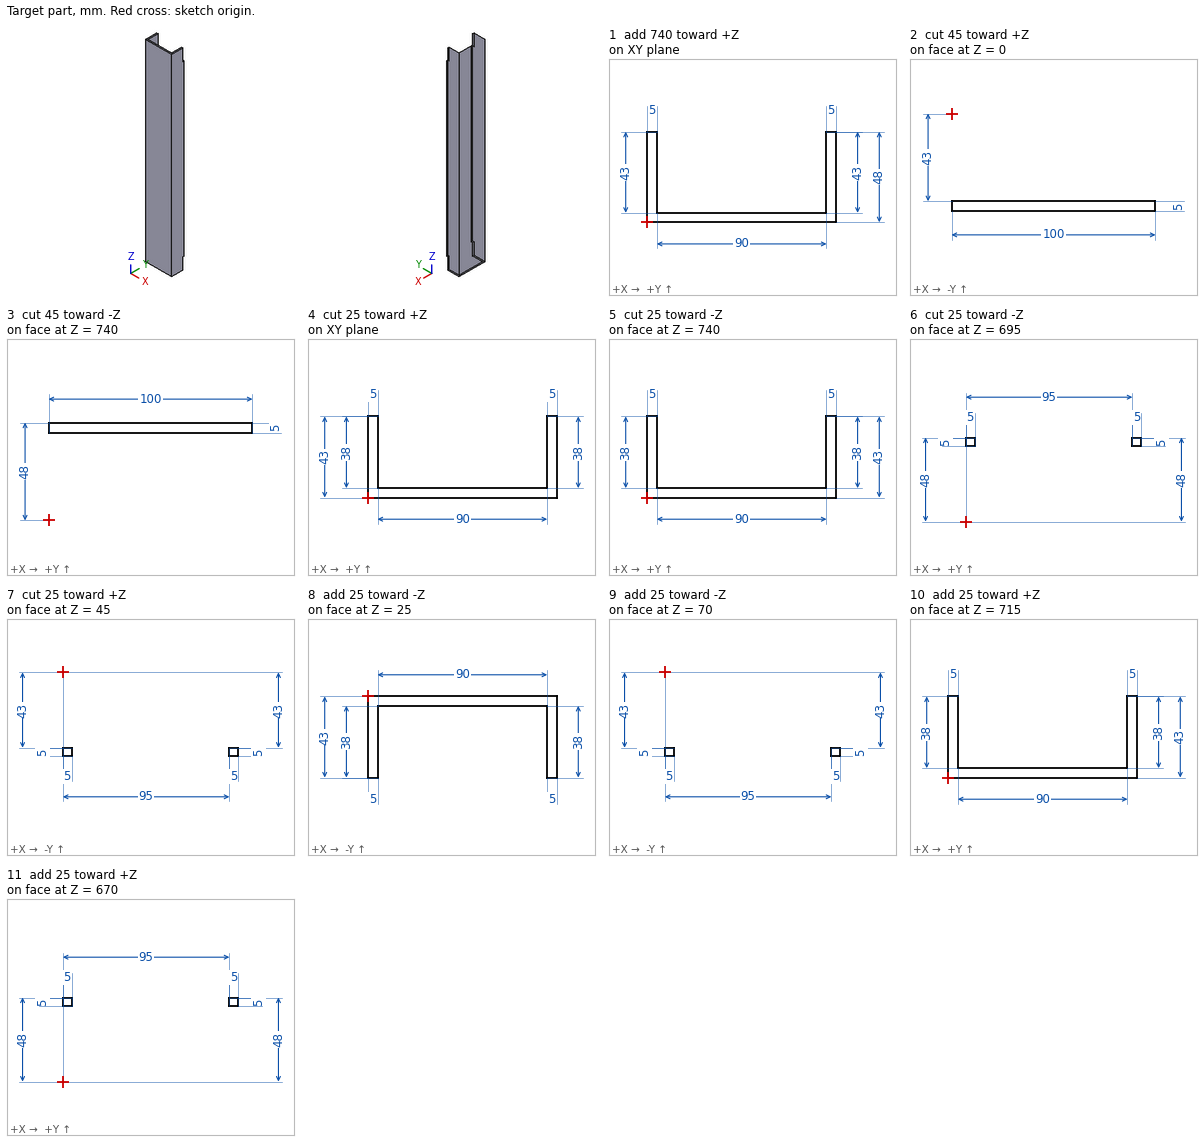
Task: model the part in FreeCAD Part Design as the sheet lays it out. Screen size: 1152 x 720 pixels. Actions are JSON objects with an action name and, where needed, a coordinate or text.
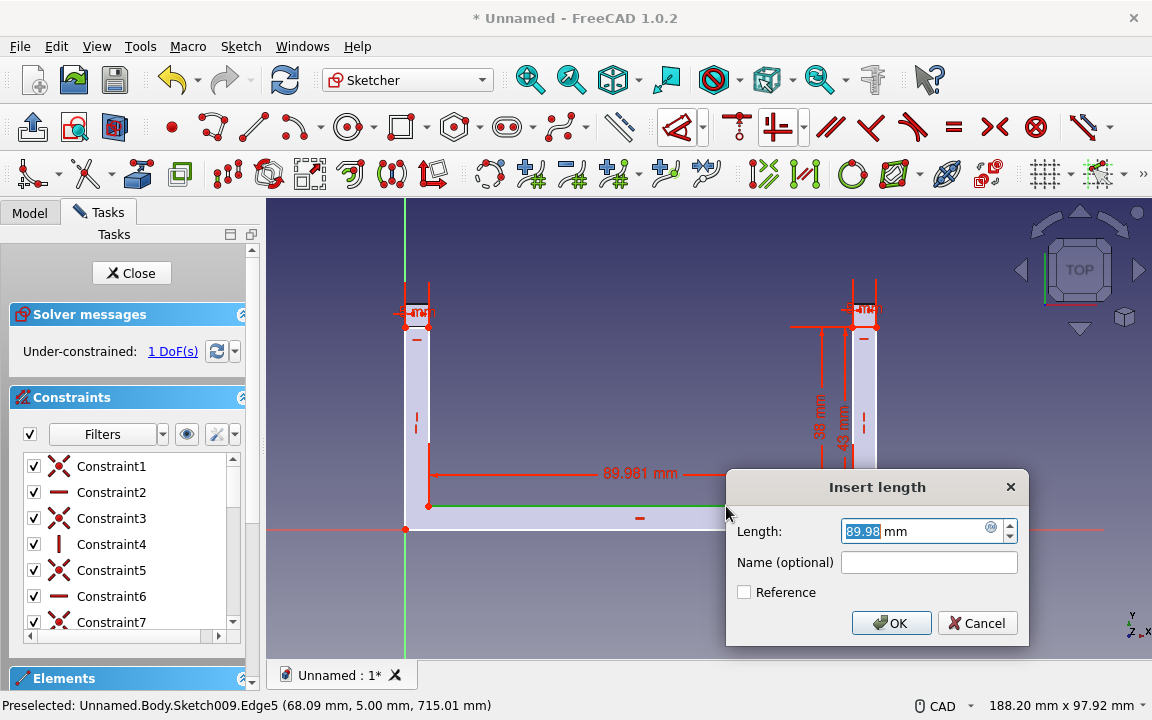
{"action": "type", "text": "90"}
{"action": "key", "text": "Return"}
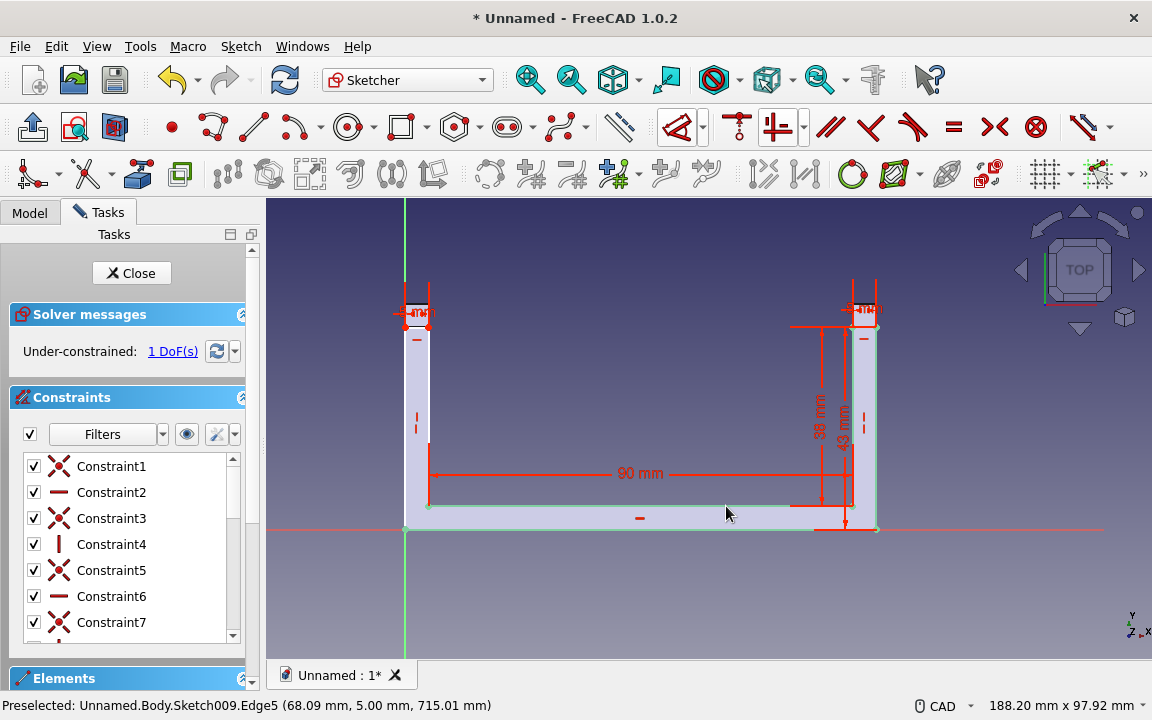
{"action": "left_click", "coordinate": [429, 453]}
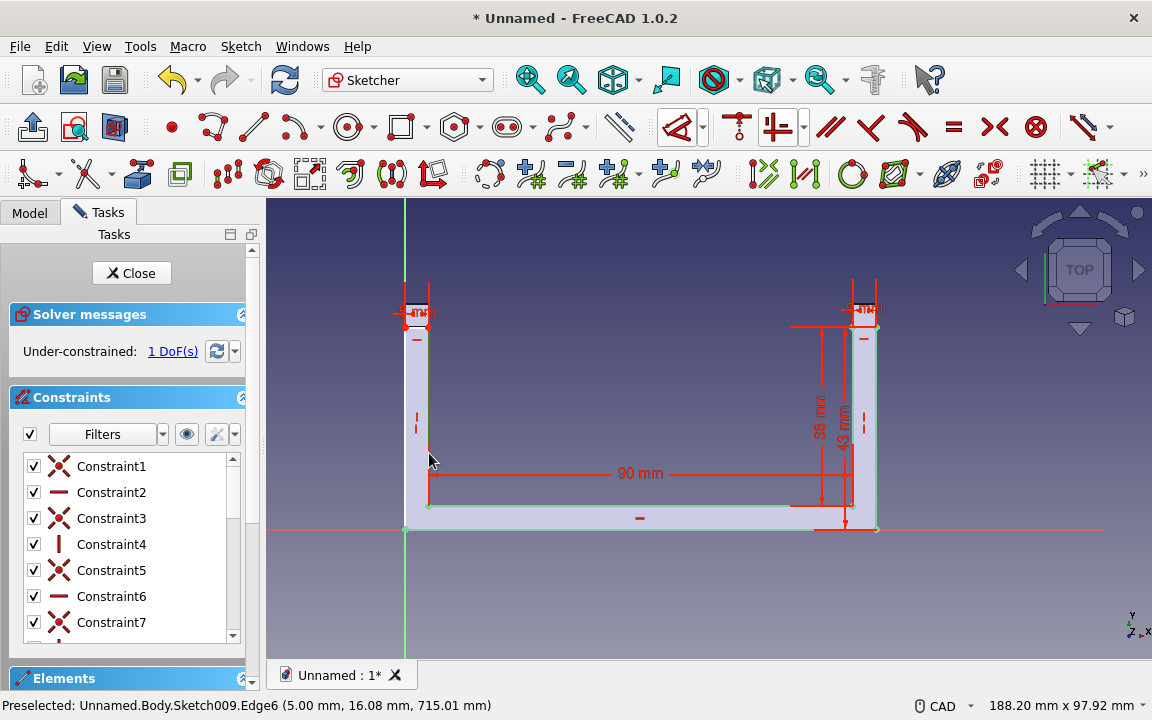
{"action": "left_click", "coordinate": [702, 128]}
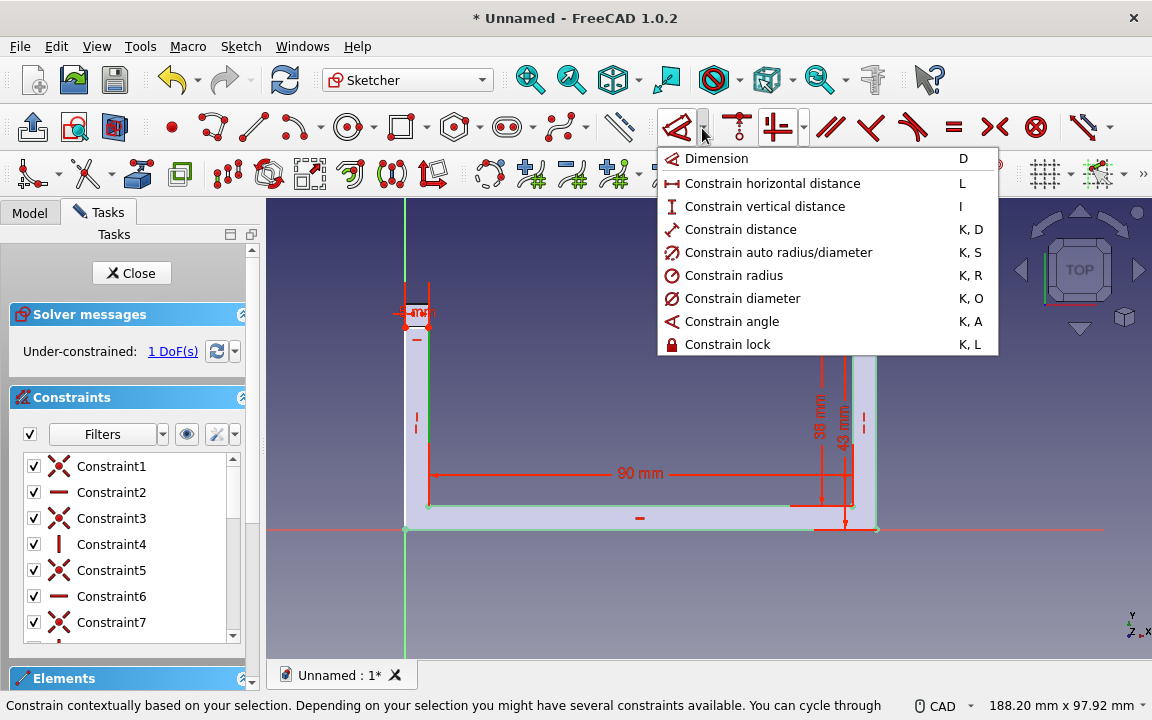
{"action": "left_click", "coordinate": [828, 206]}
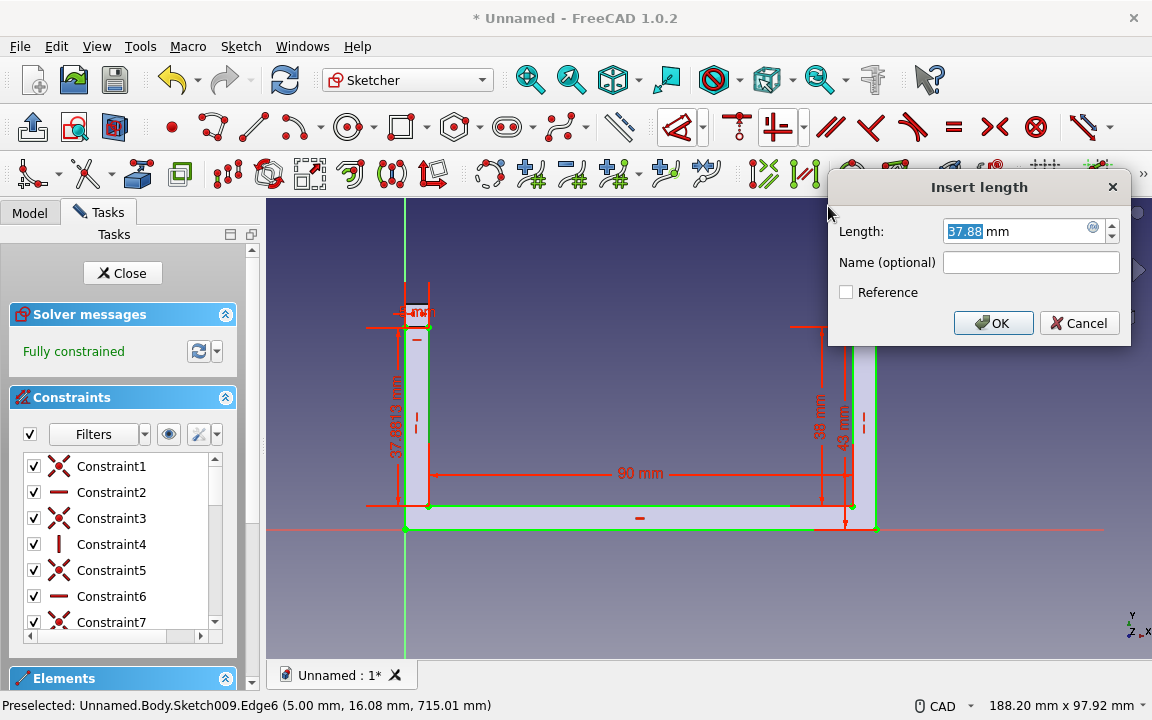
{"action": "type", "text": "38"}
{"action": "key", "text": "Return"}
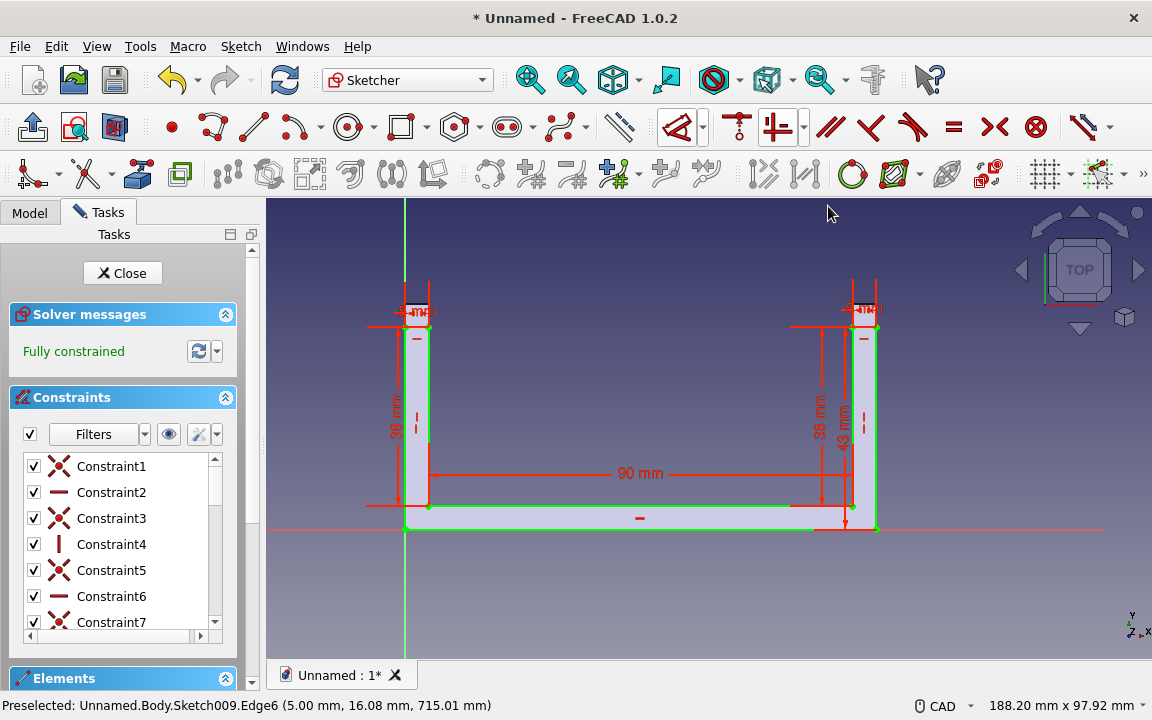
{"action": "left_click", "coordinate": [123, 273]}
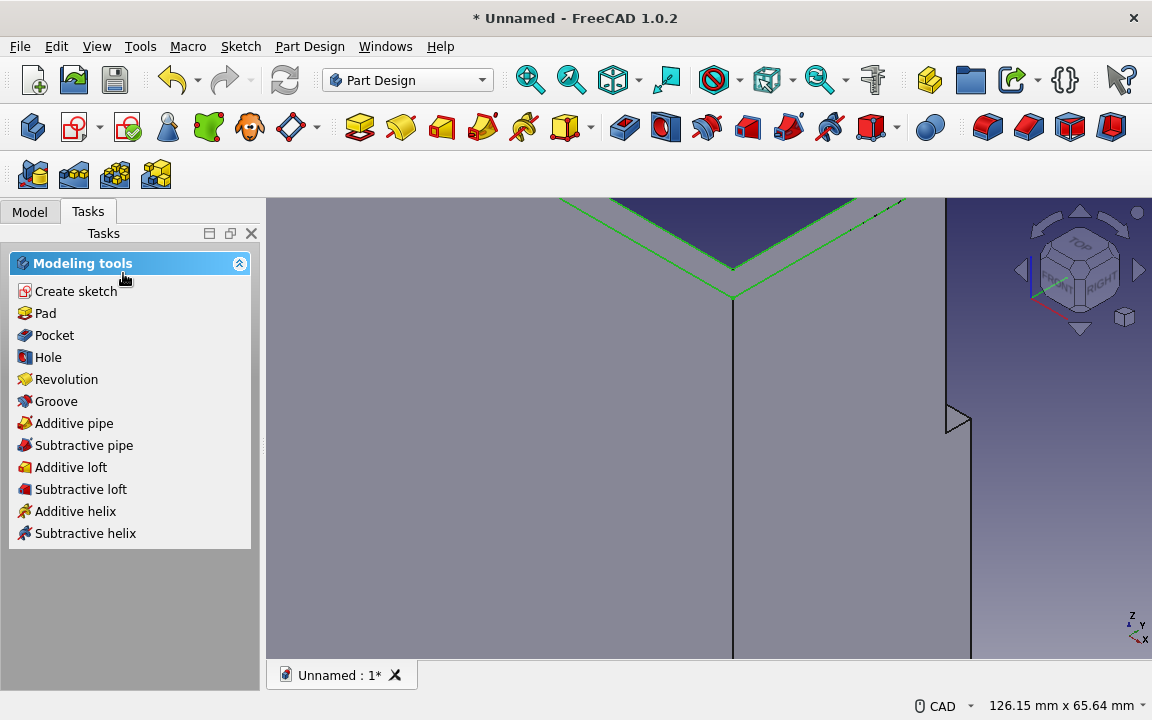
{"action": "left_click", "coordinate": [360, 128]}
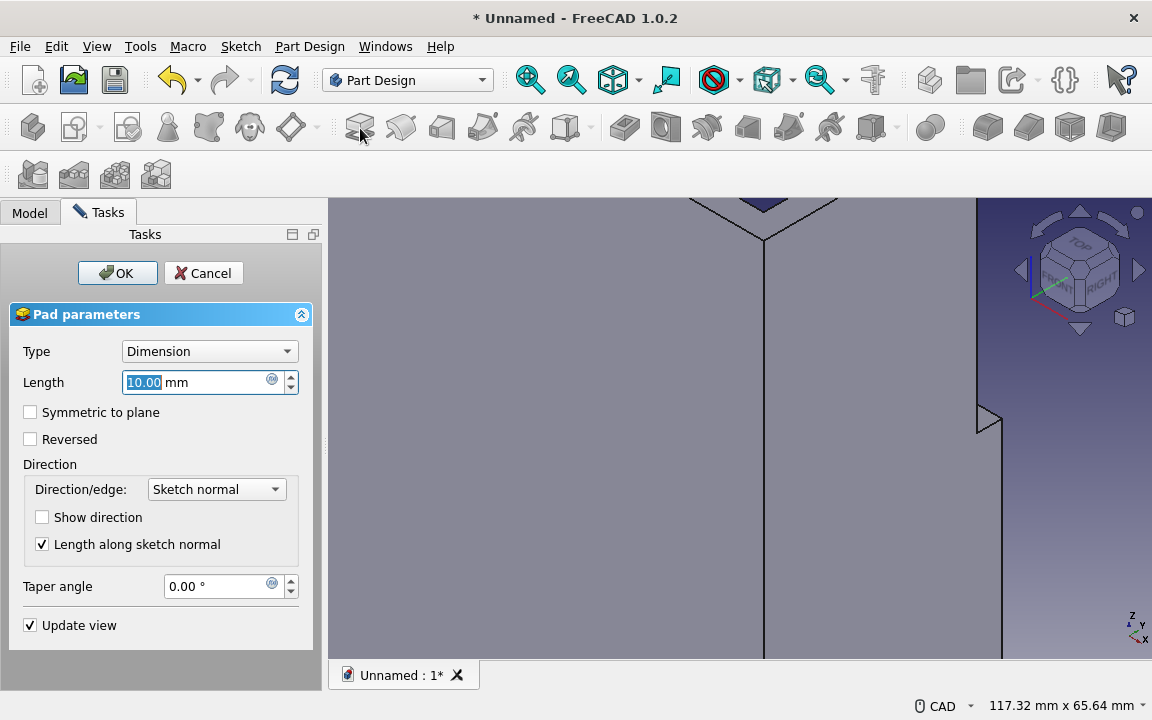
{"action": "type", "text": "25"}
{"action": "key", "text": "Tab"}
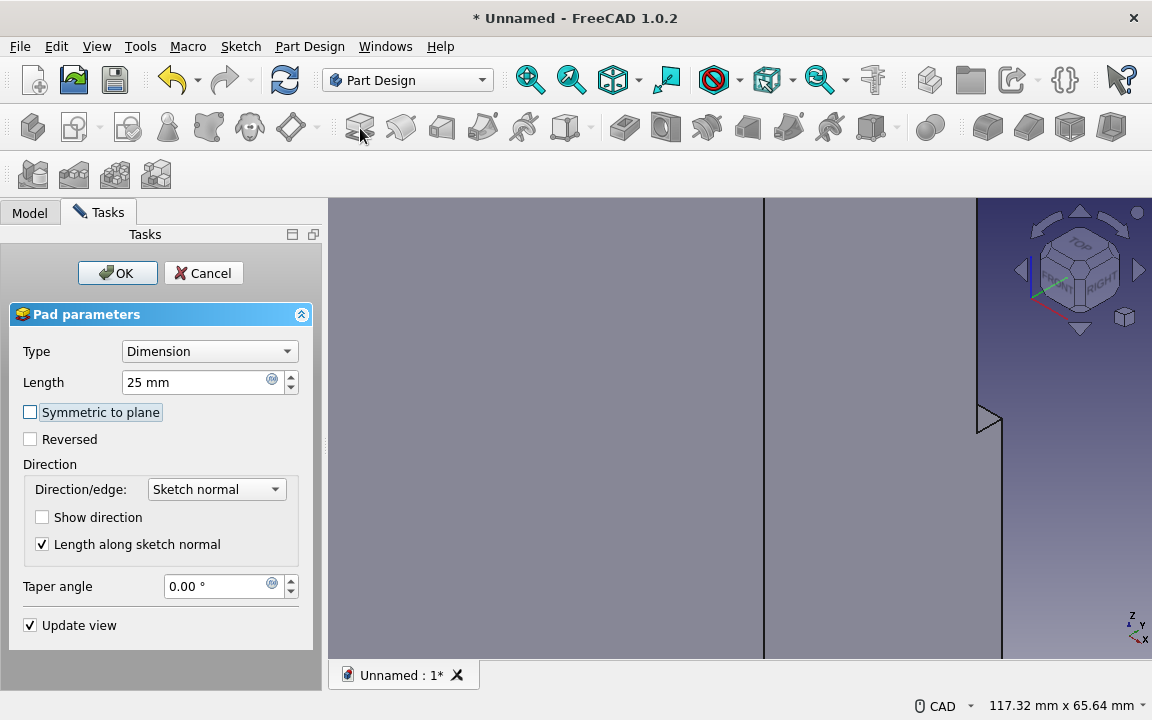
{"action": "left_click", "coordinate": [118, 273]}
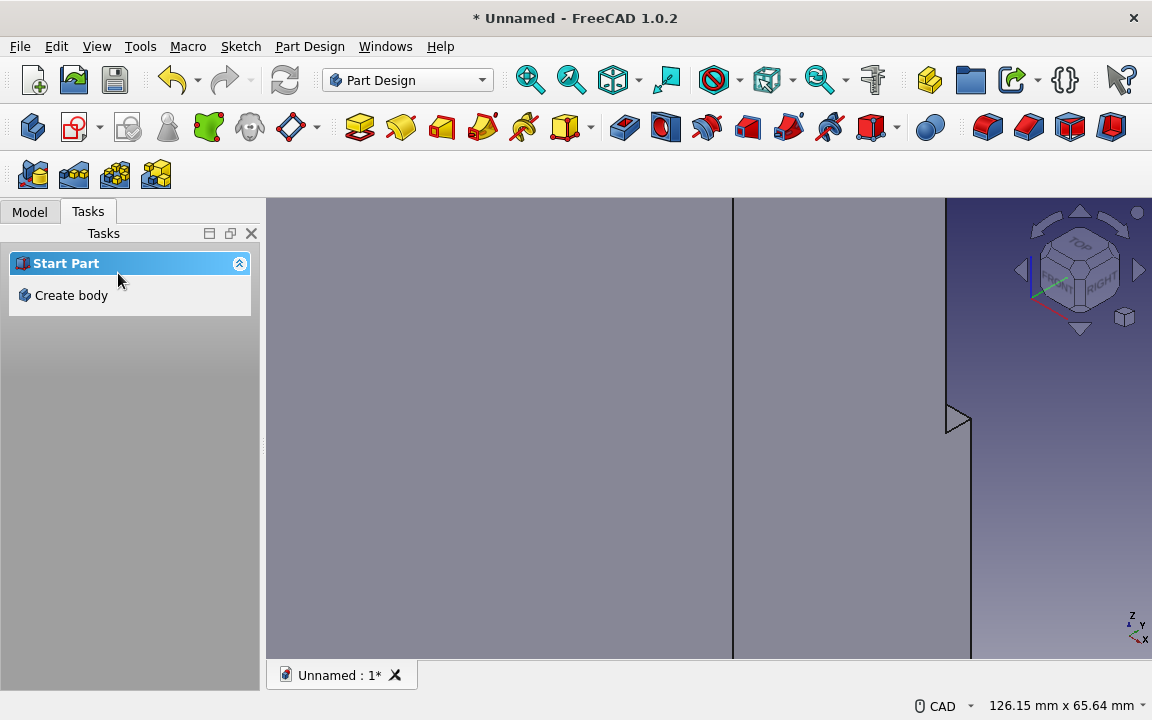
{"action": "left_click", "coordinate": [531, 80]}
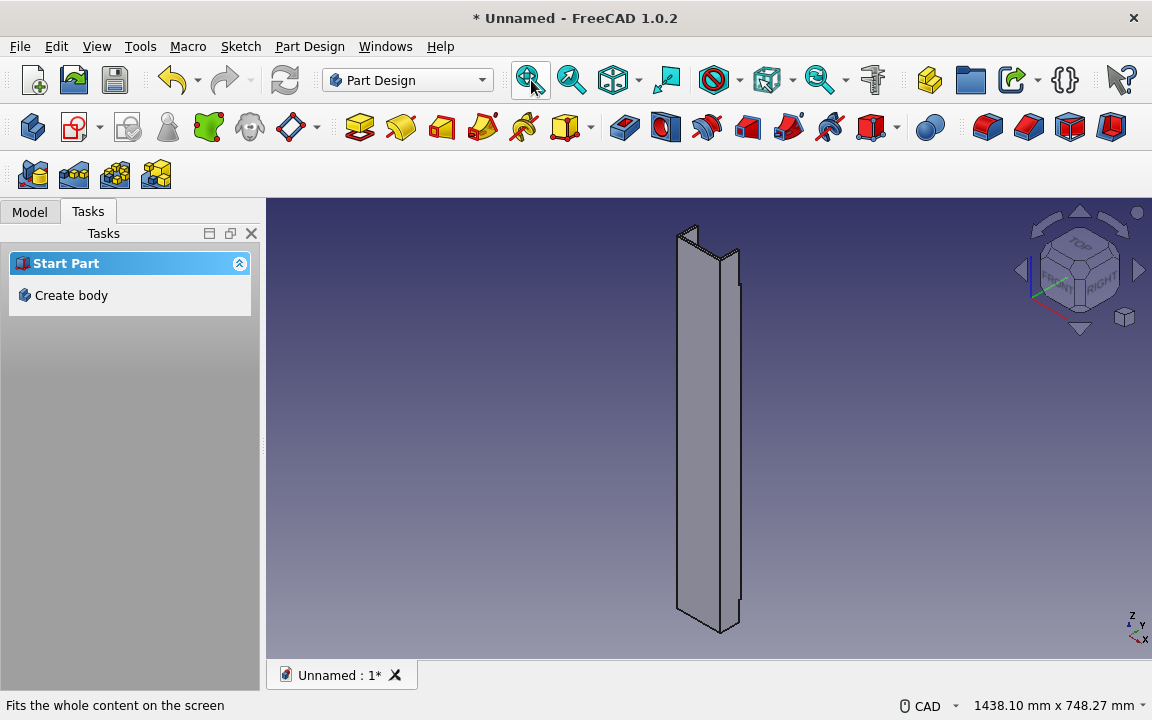
{"action": "scroll", "coordinate": [698, 259], "scroll_direction": "up", "scroll_amount": 11}